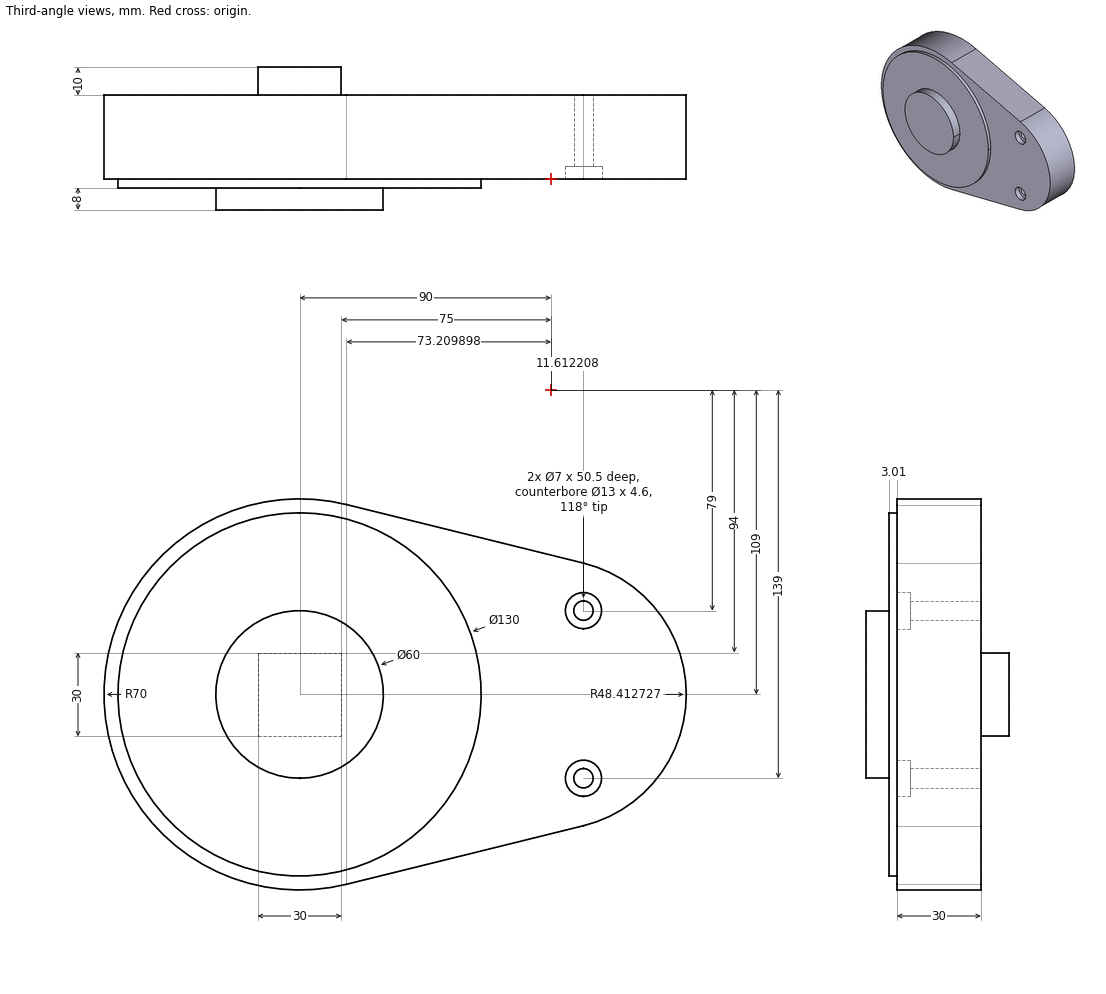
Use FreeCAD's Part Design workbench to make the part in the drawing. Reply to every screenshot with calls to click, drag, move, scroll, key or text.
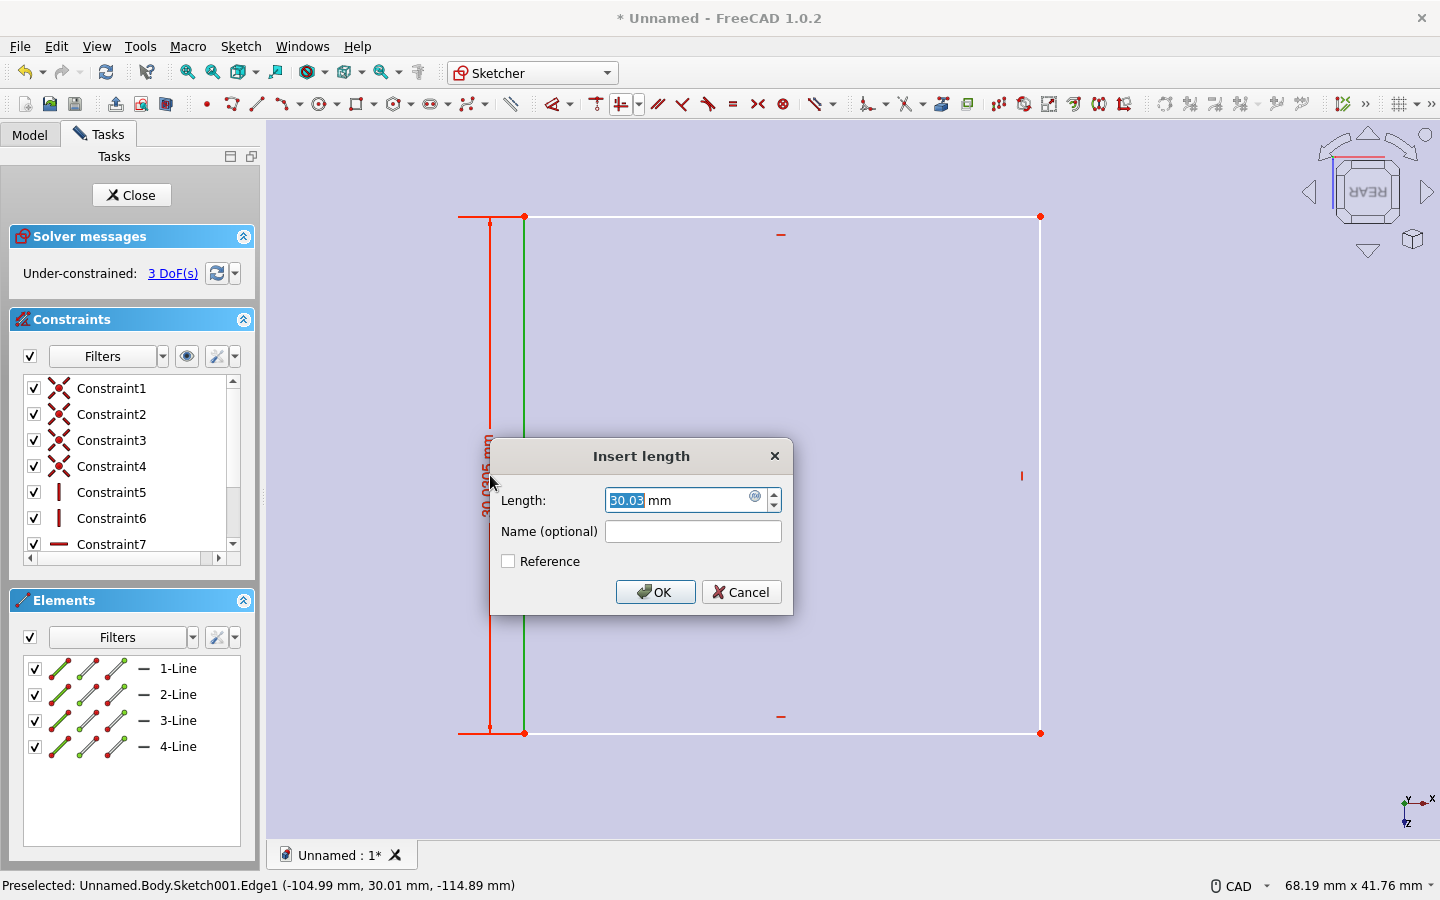
text(30)
key(Return)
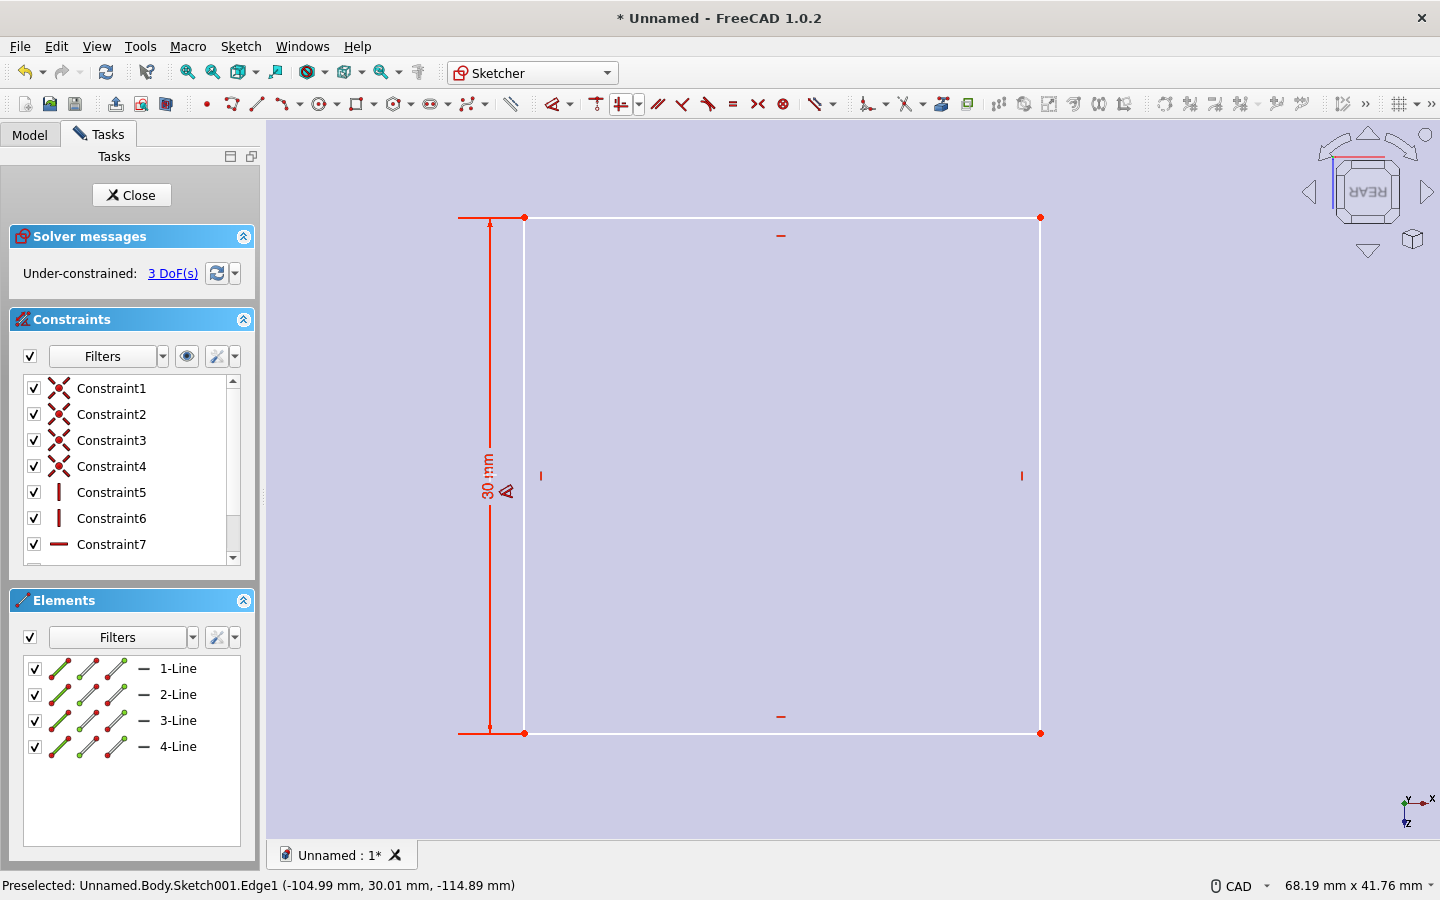
click(679, 734)
click(782, 768)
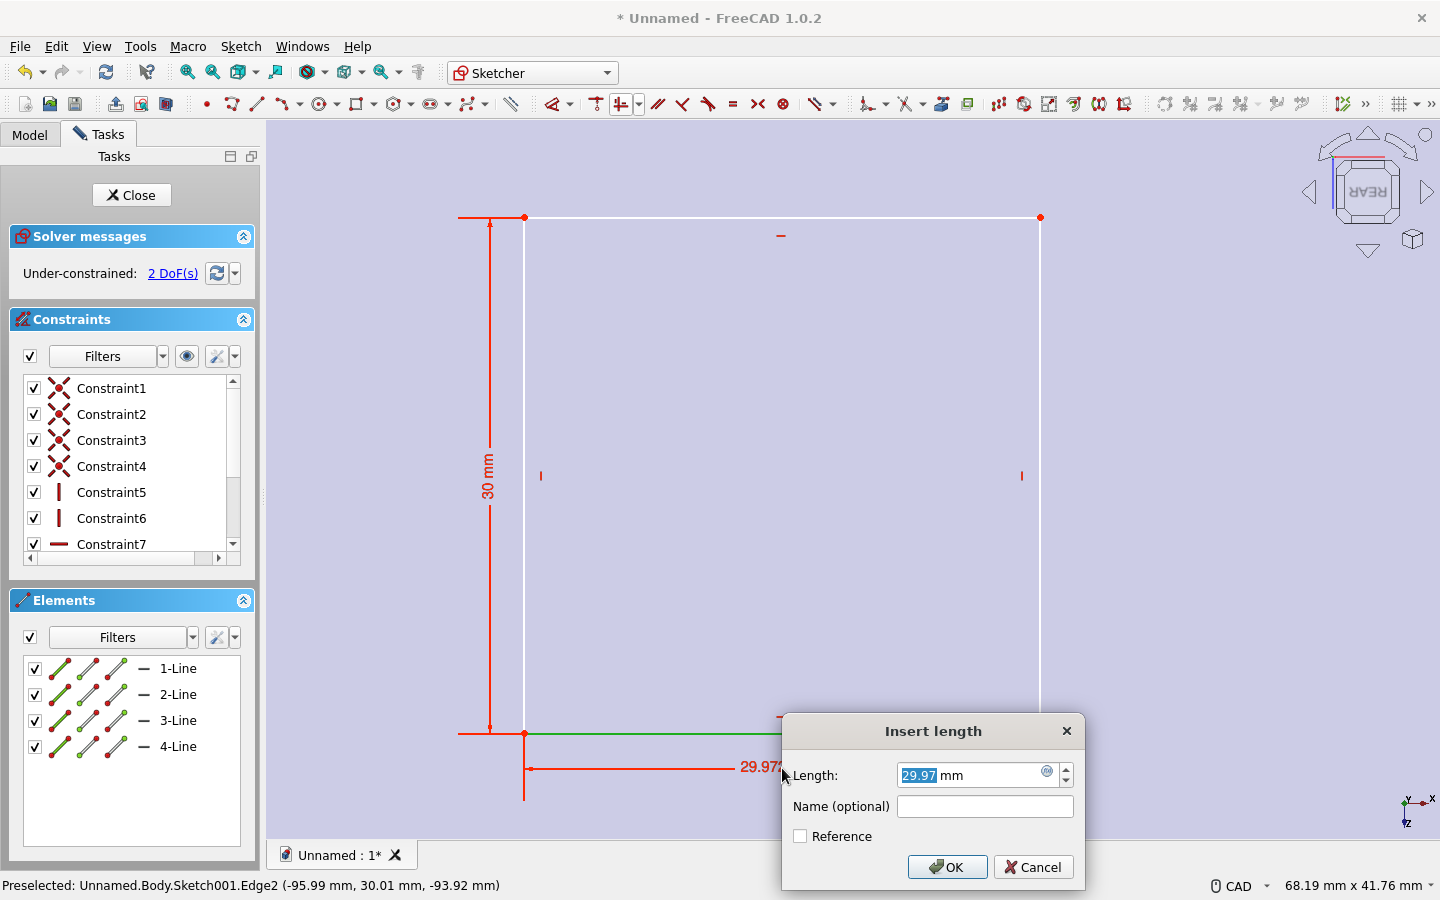
text(30)
key(Return)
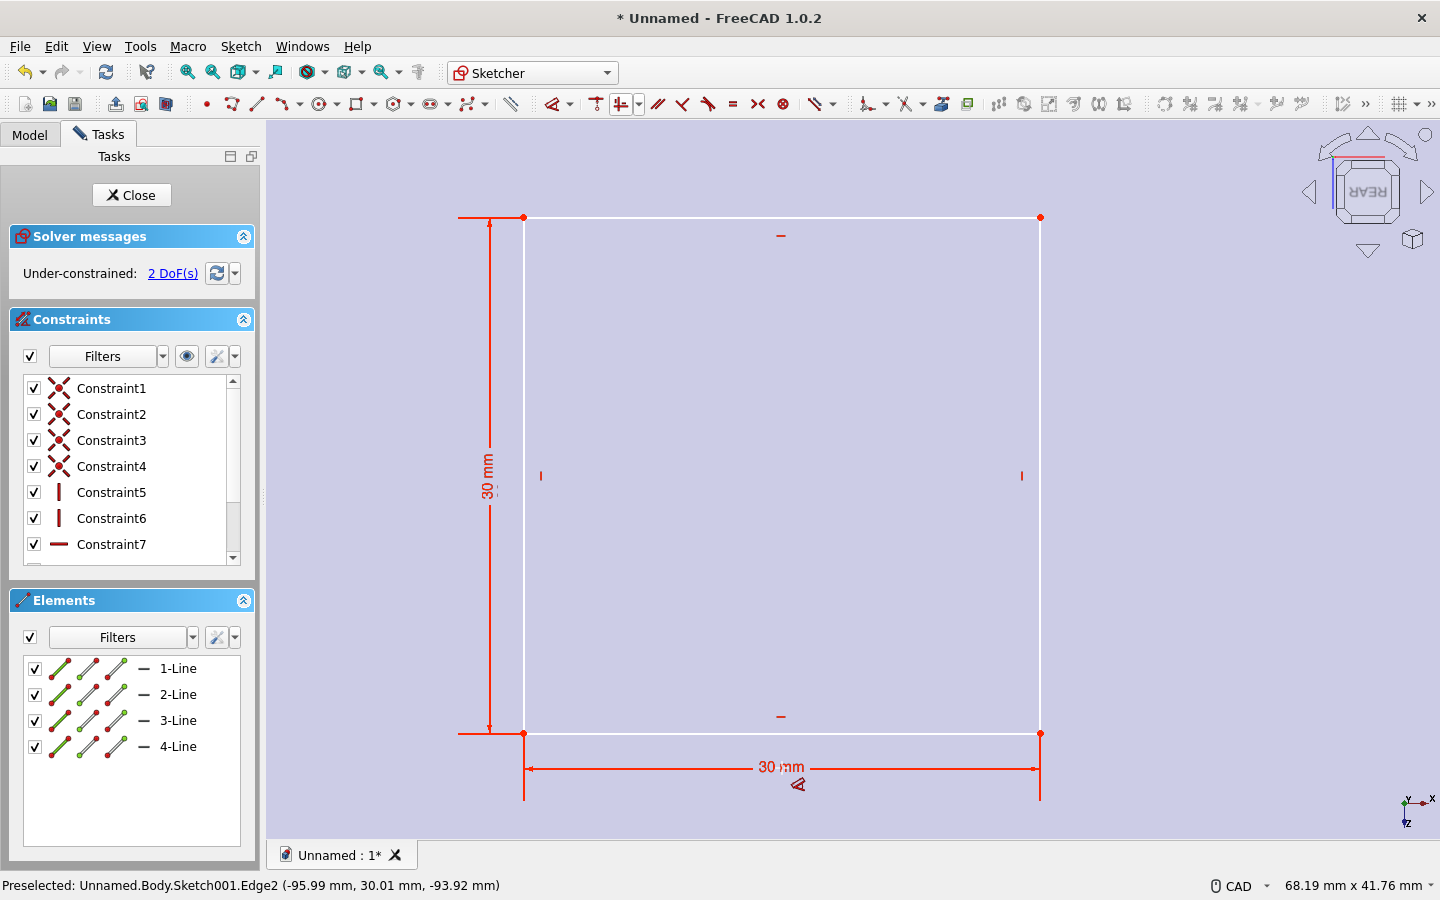
click(524, 734)
click(490, 772)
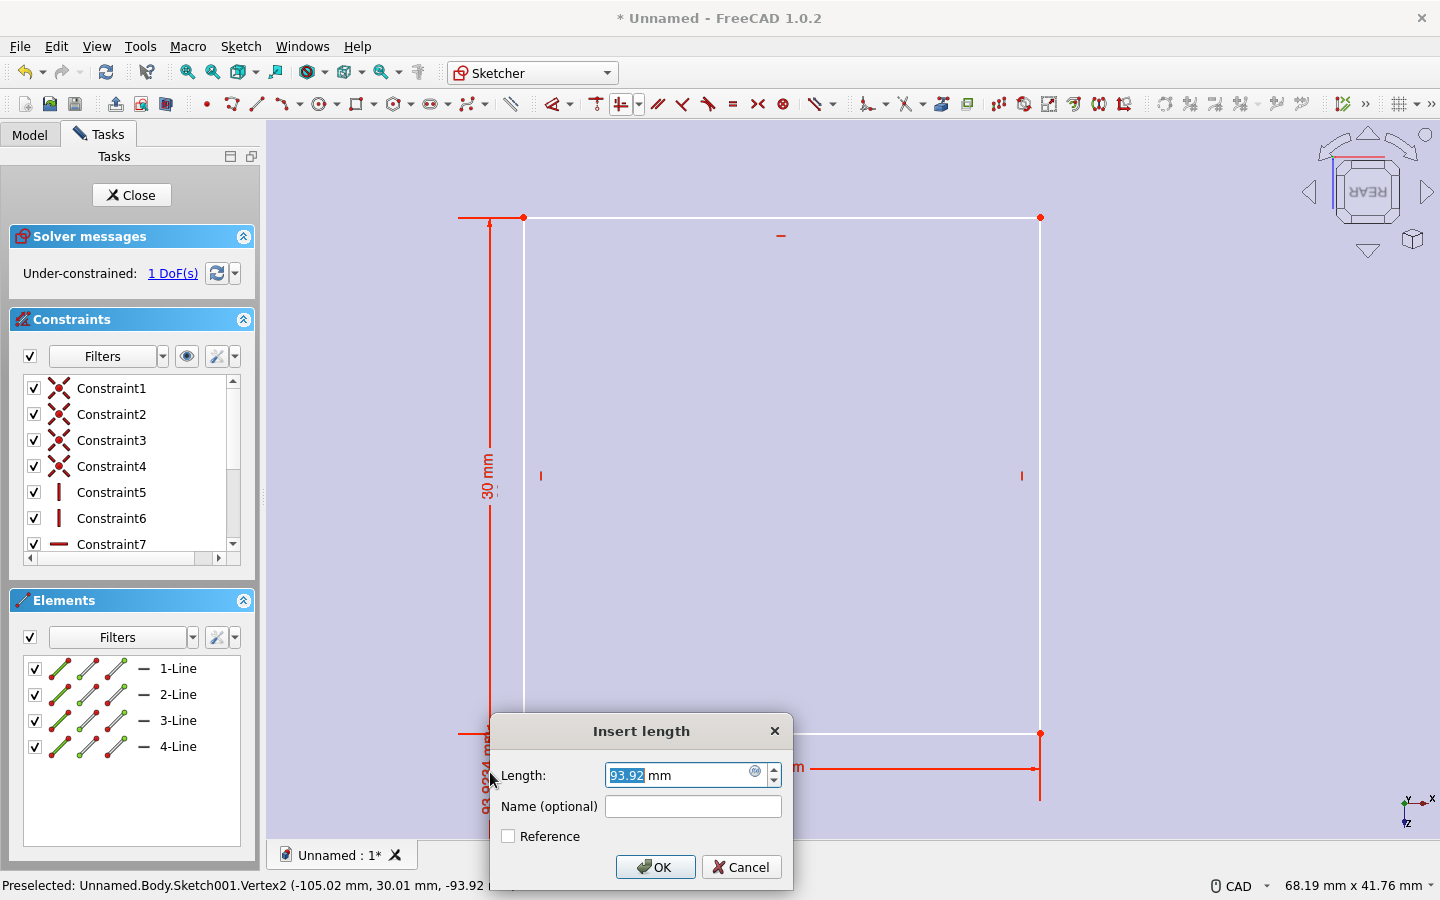
text(94)
key(Return)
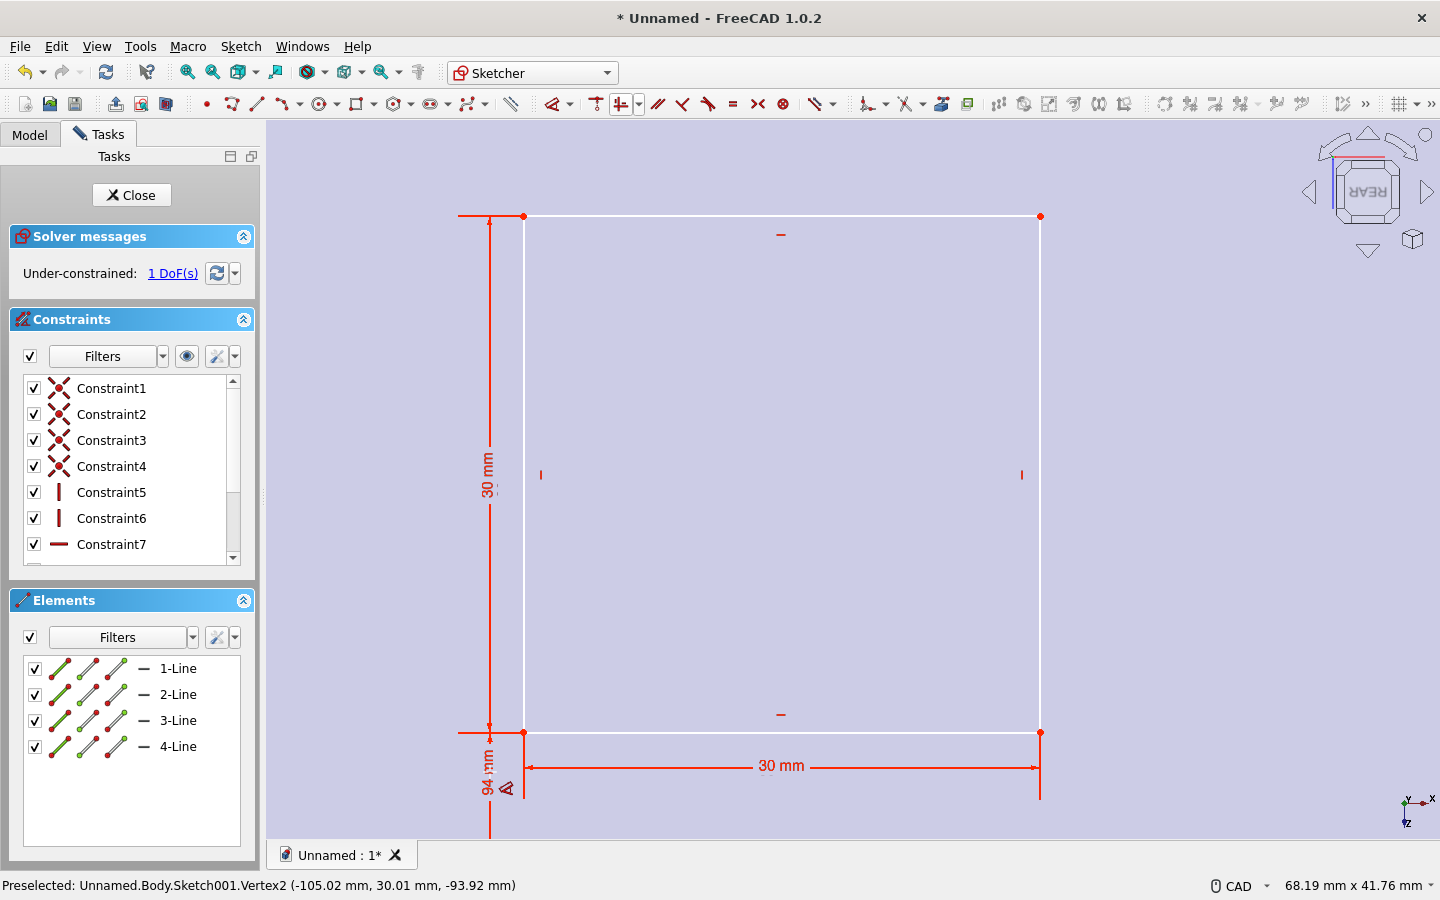
click(1040, 733)
click(1157, 699)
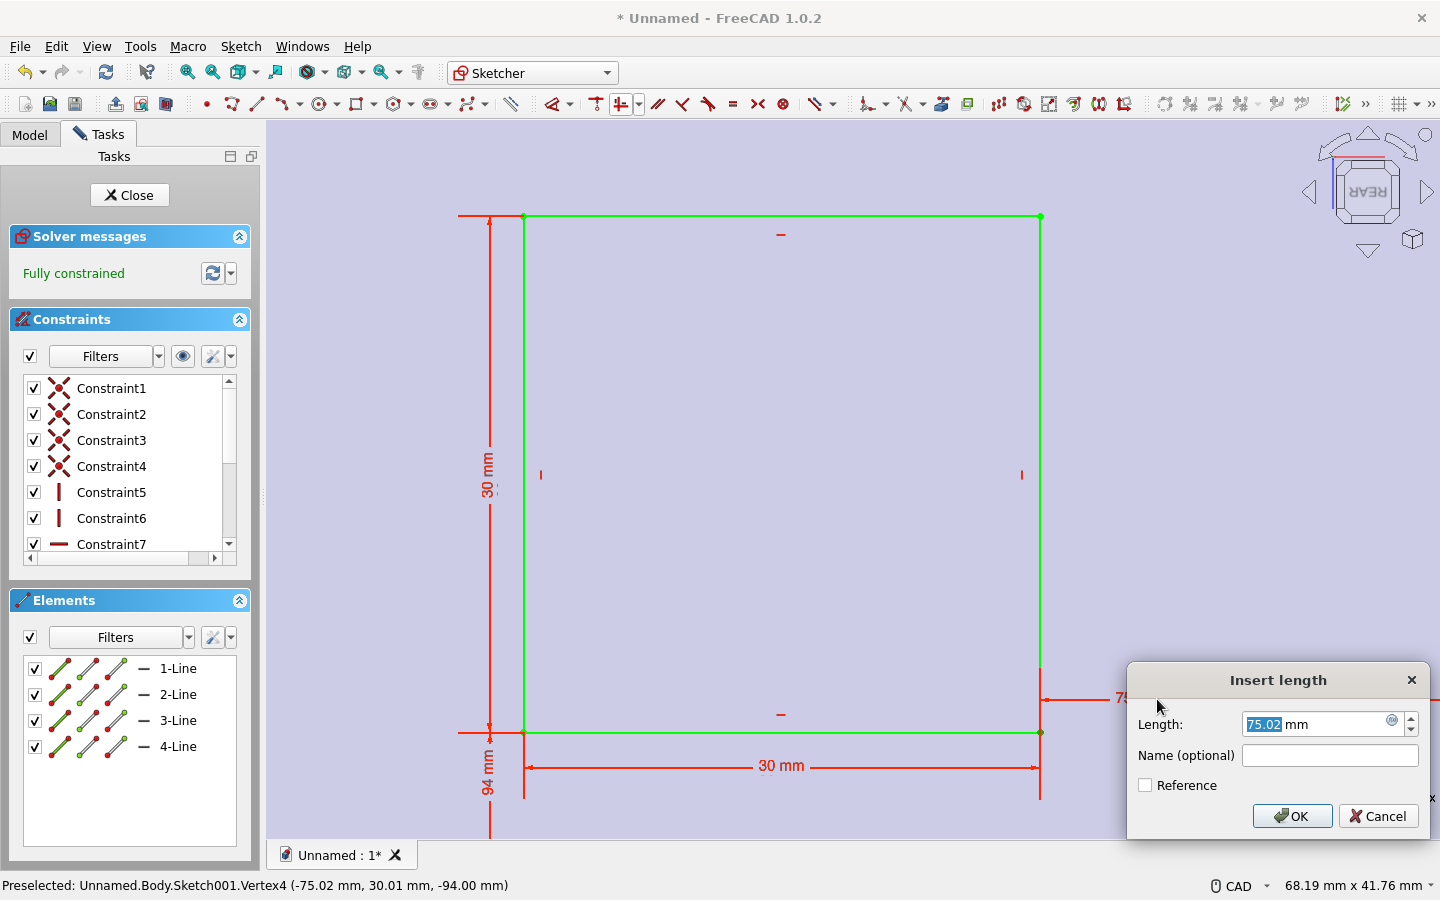
text(75)
key(Return)
key(Escape)